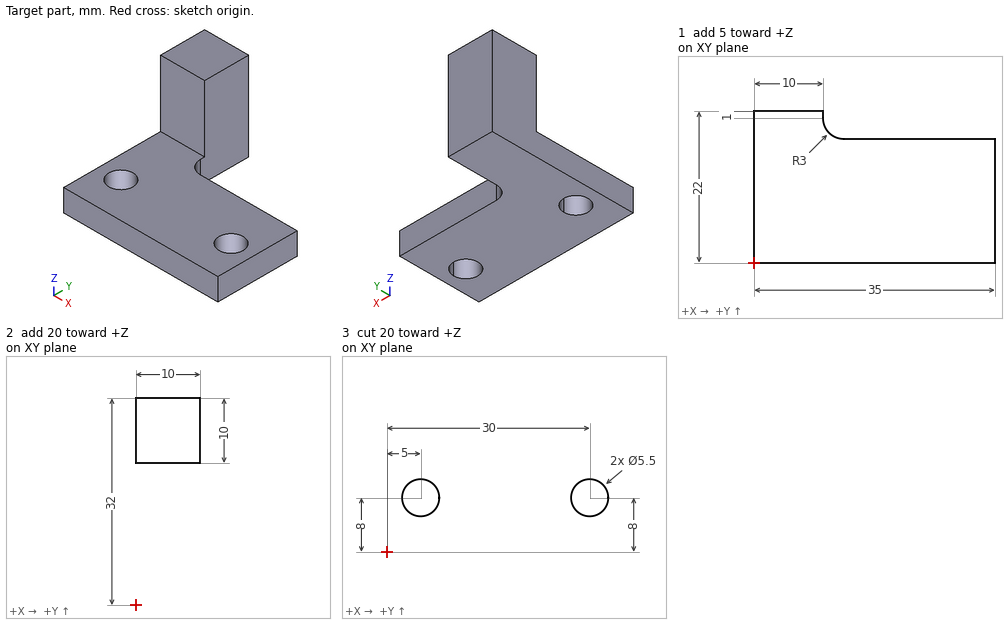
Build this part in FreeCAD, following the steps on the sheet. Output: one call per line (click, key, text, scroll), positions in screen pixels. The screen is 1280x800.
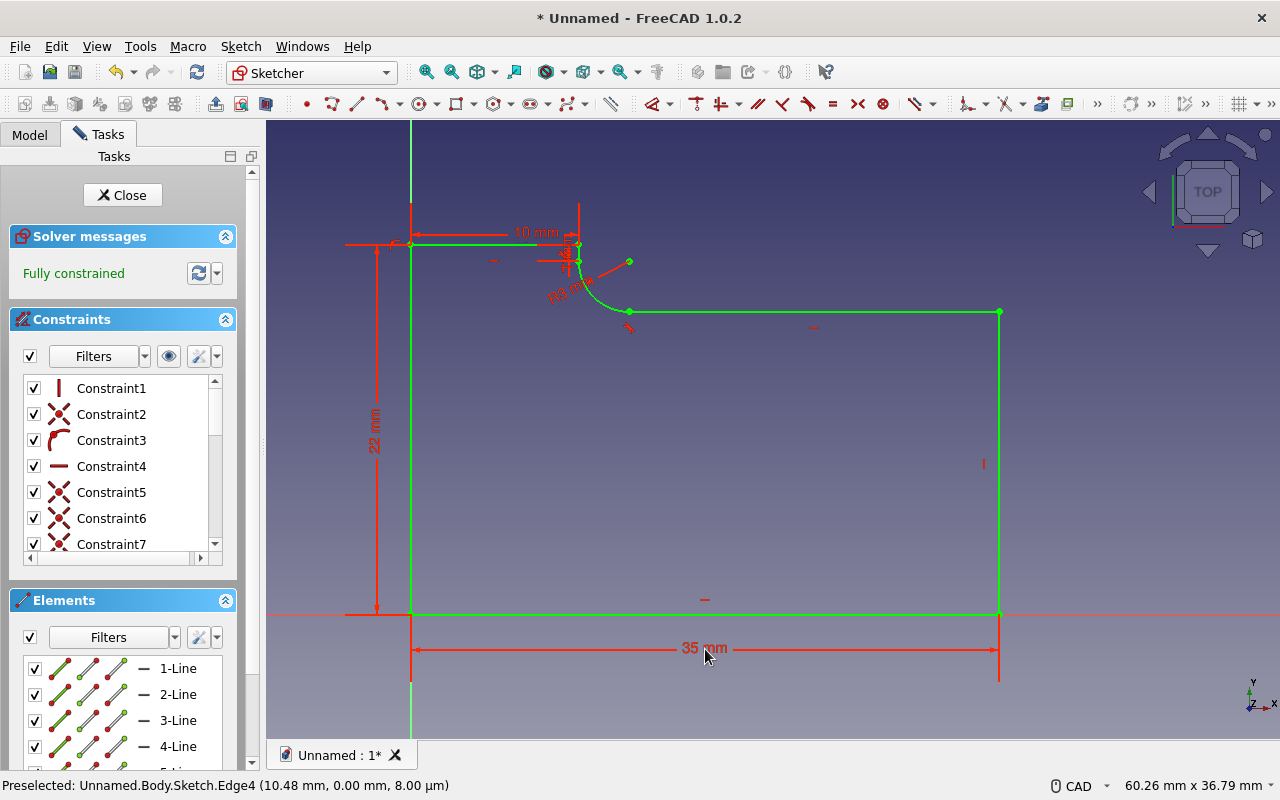
click(123, 195)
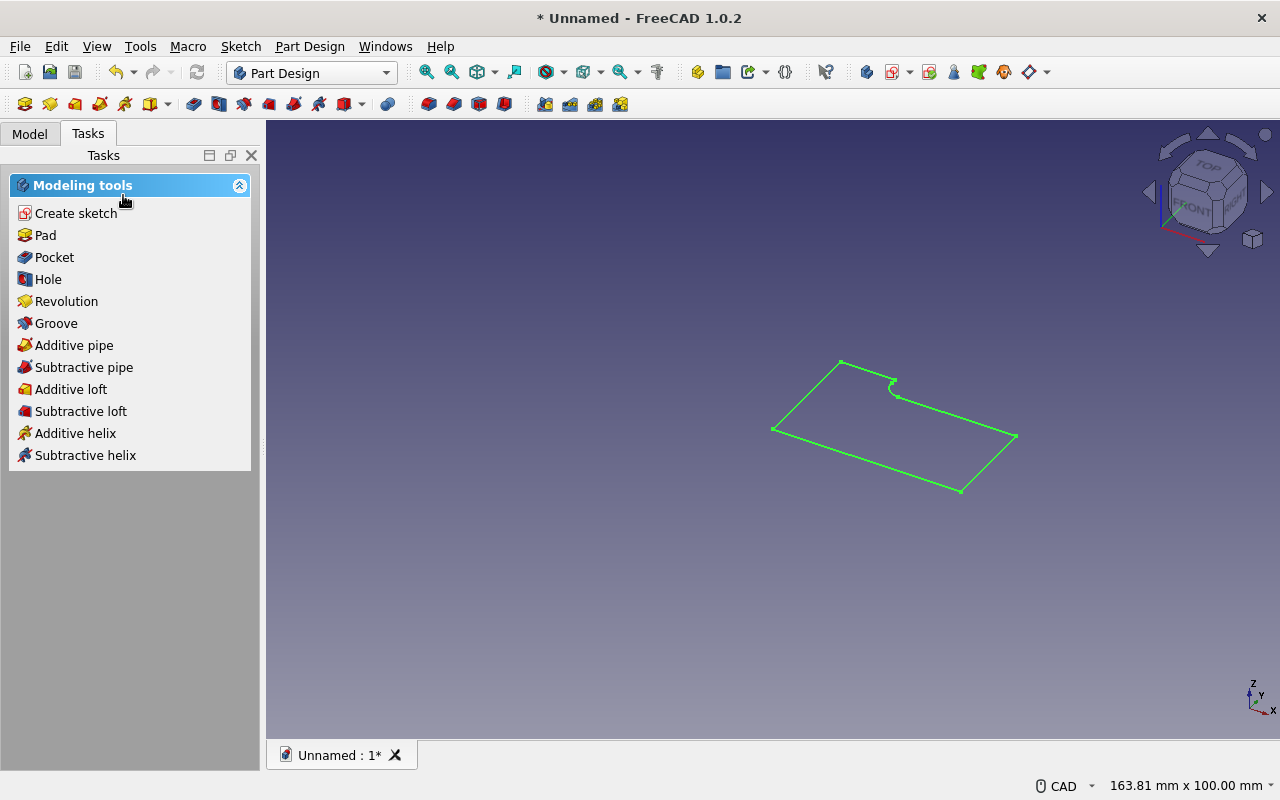
click(25, 104)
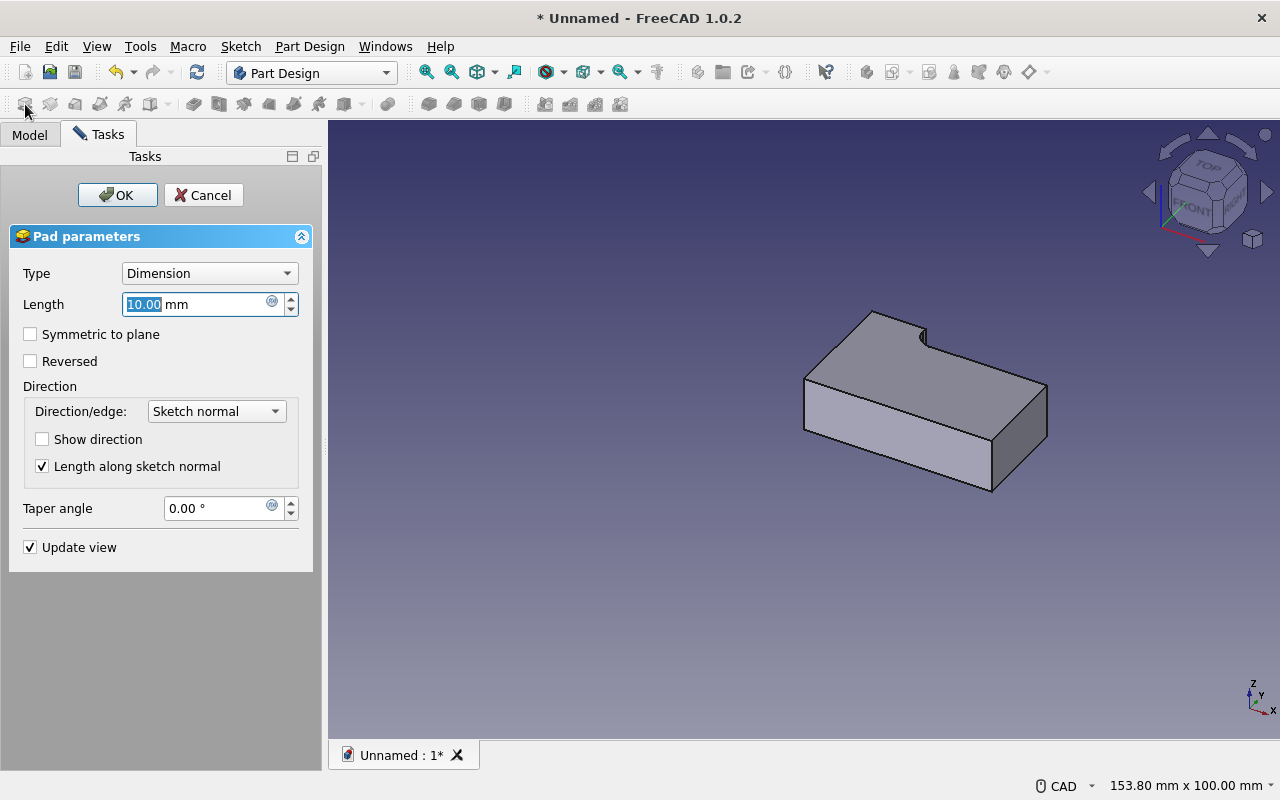
text(5)
key(Tab)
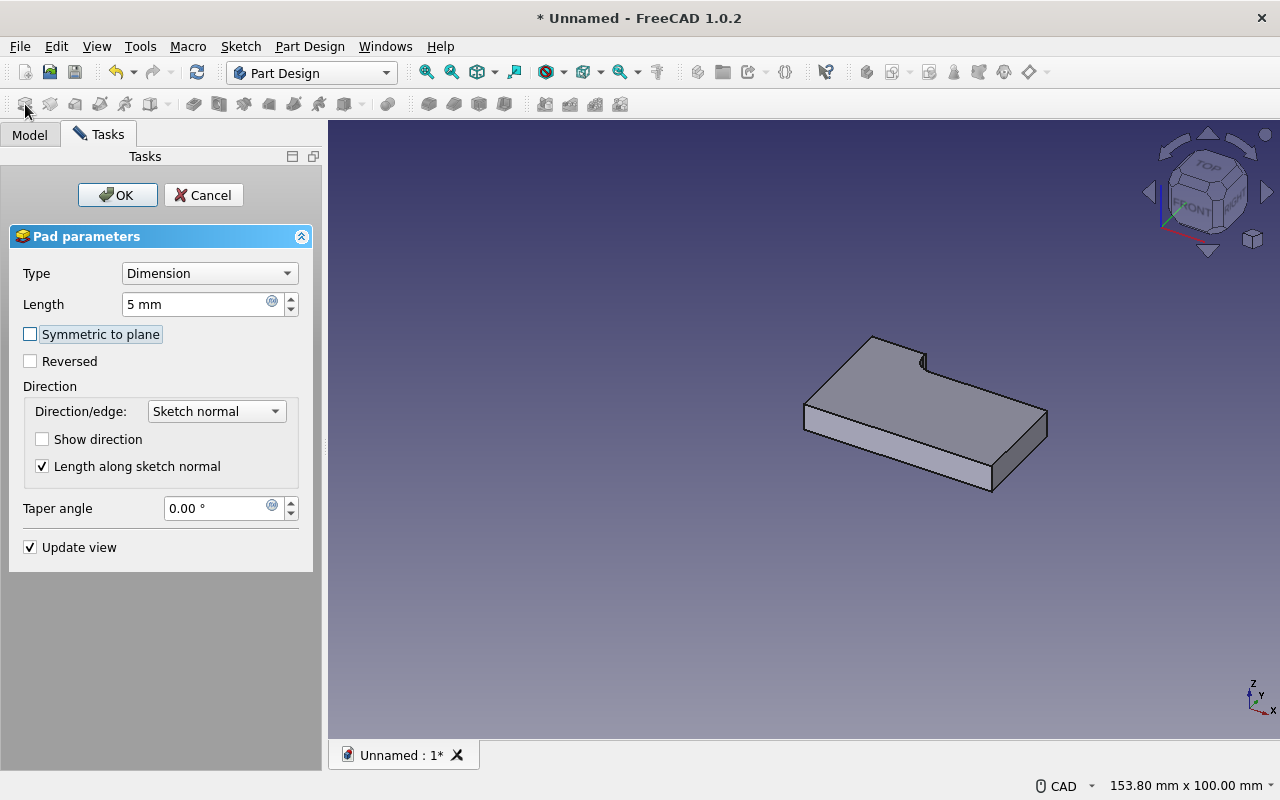
click(118, 195)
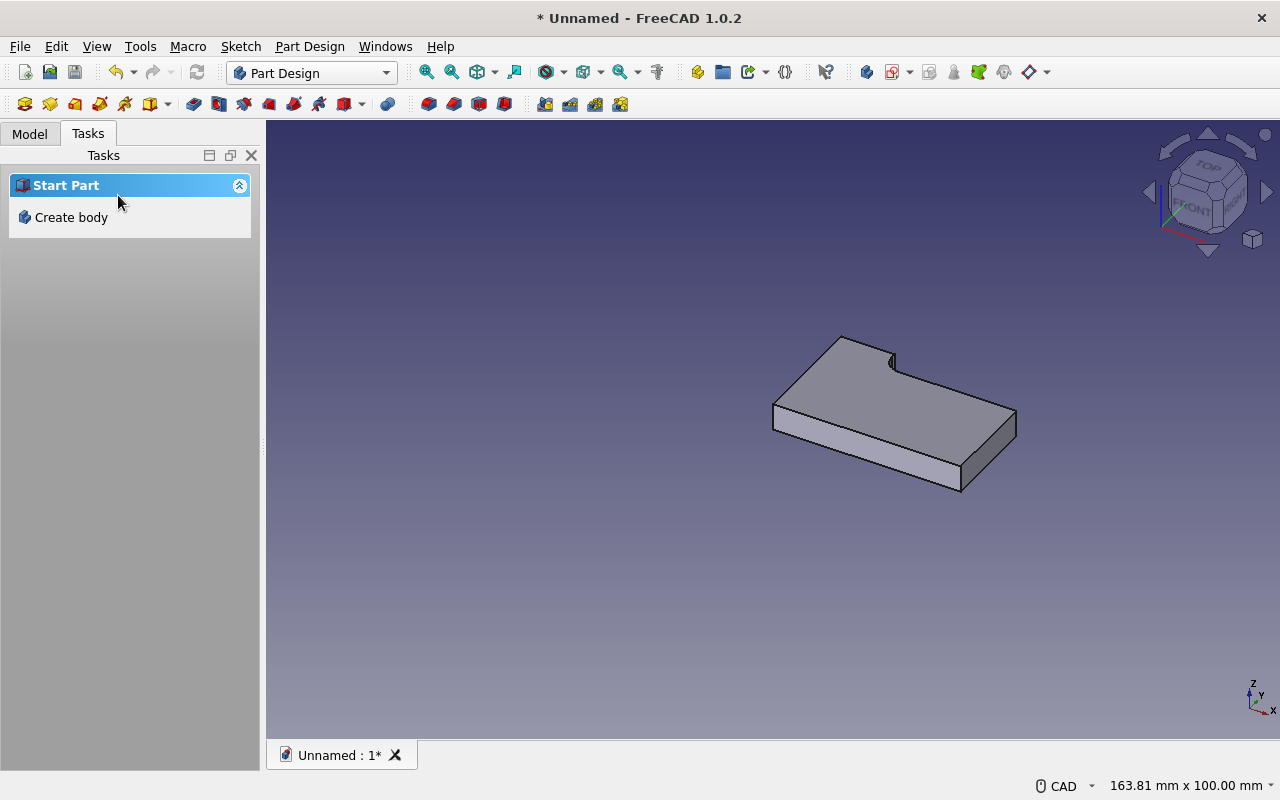
click(427, 72)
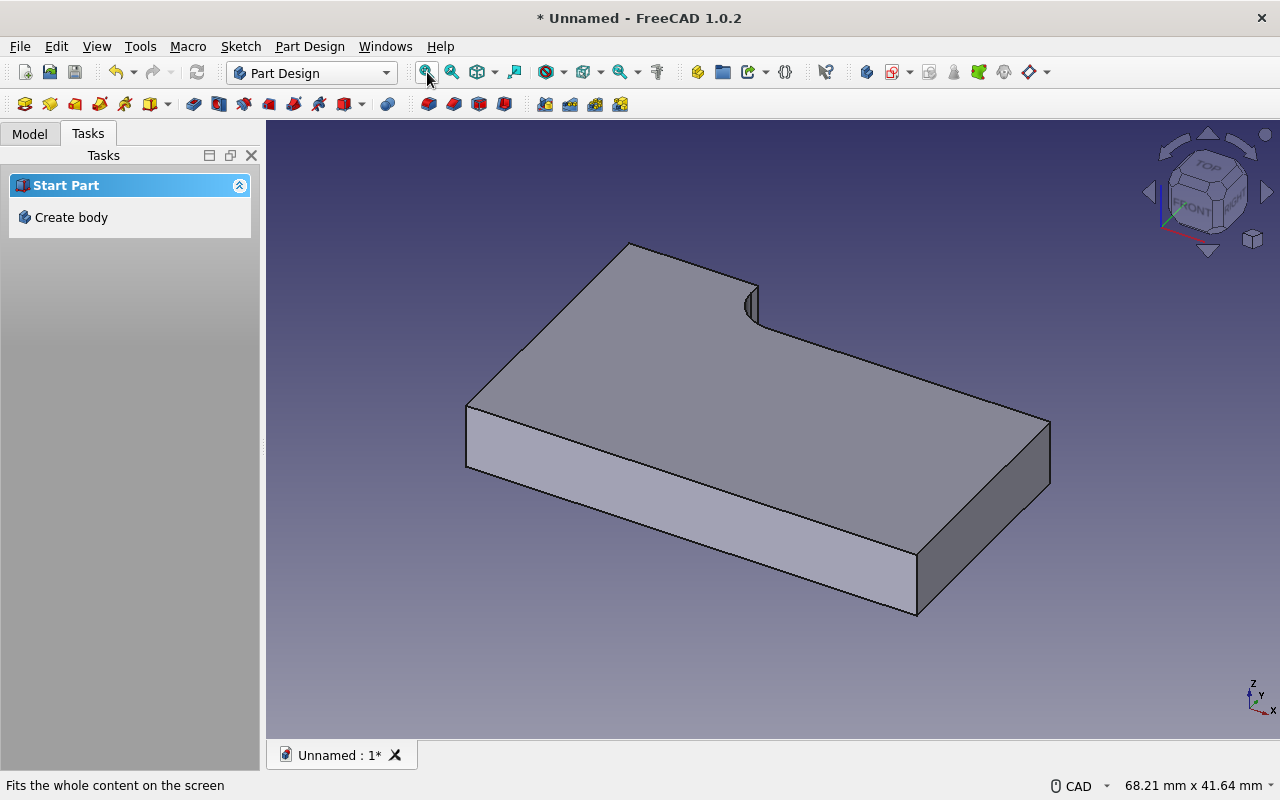
click(892, 72)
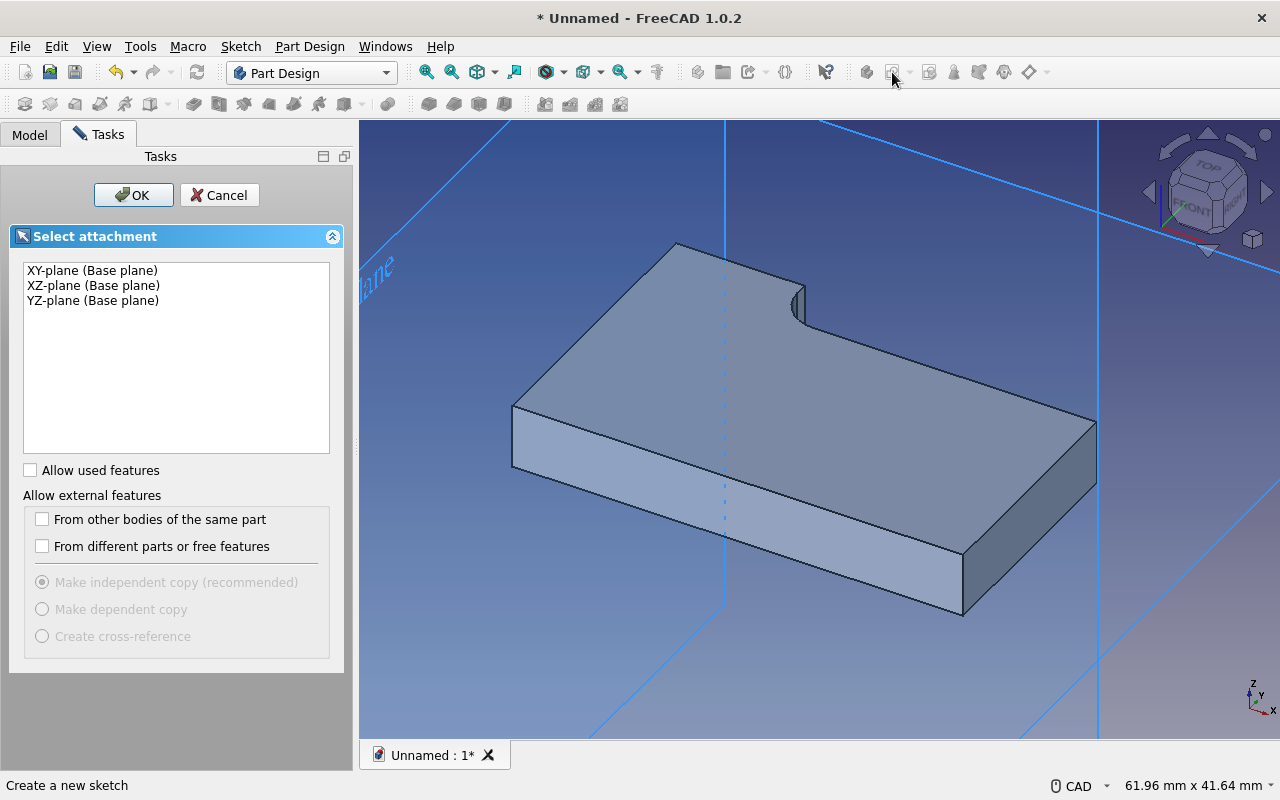
click(84, 270)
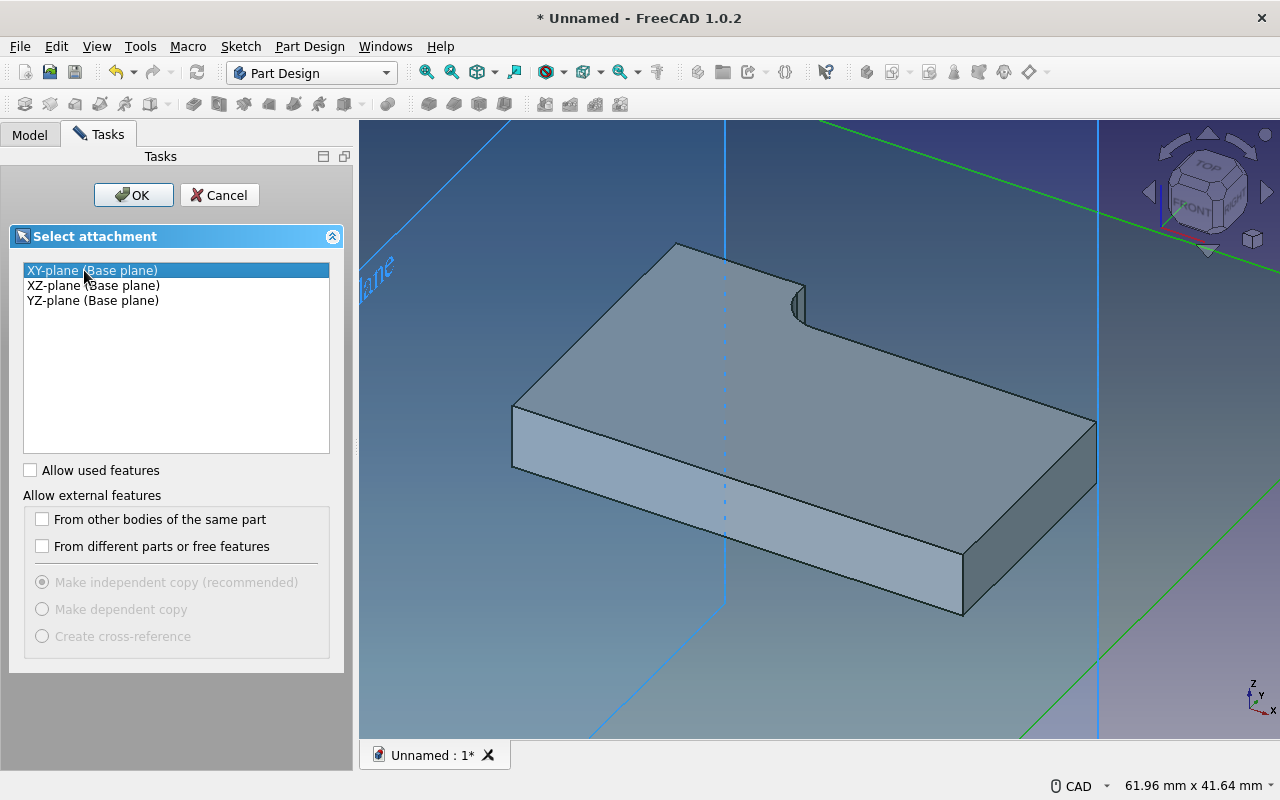
click(134, 195)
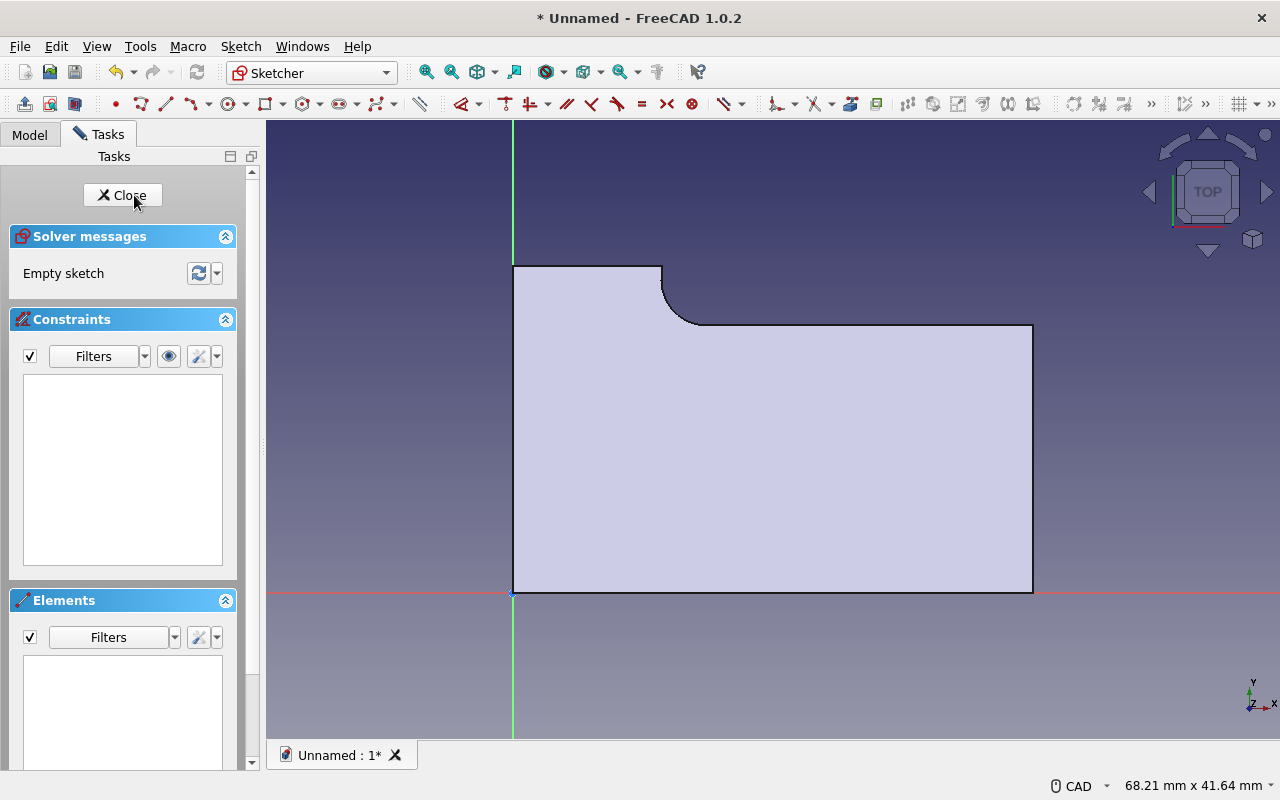
click(75, 104)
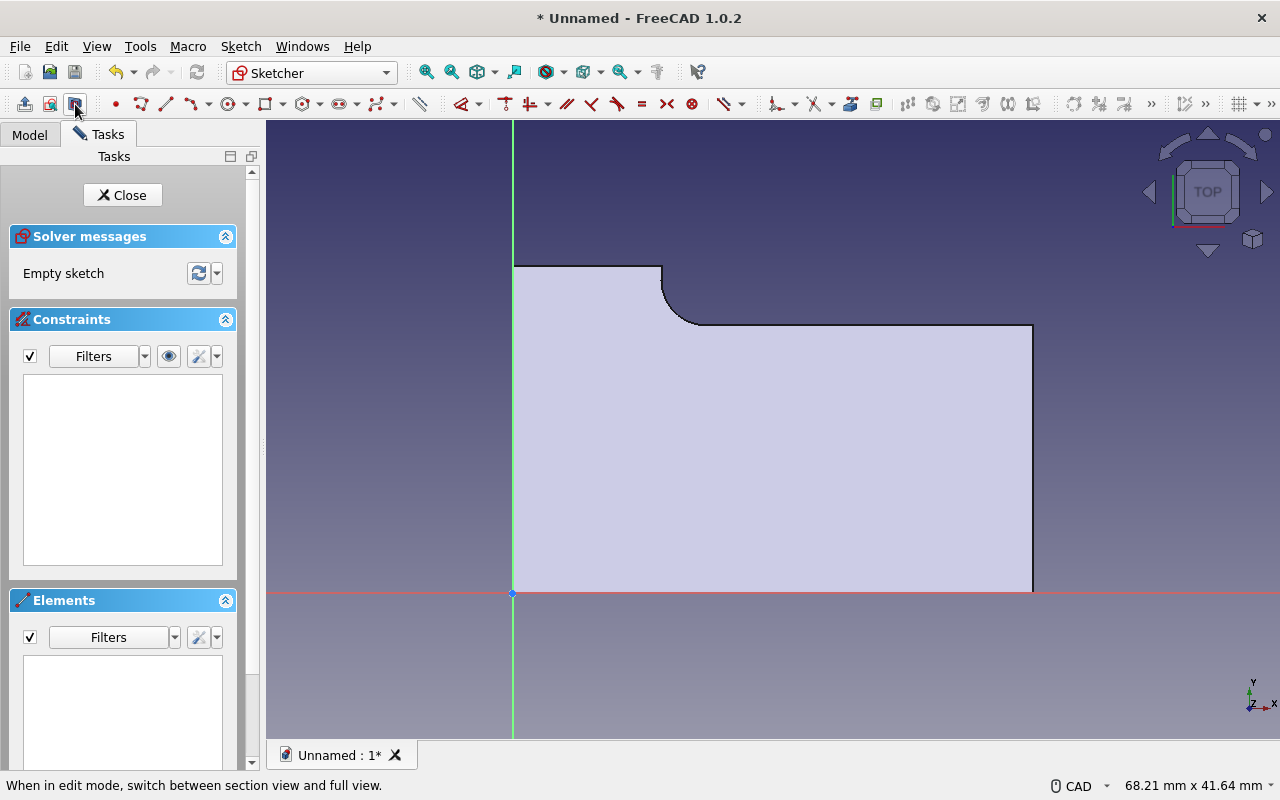
scroll(704, 430, down, 5)